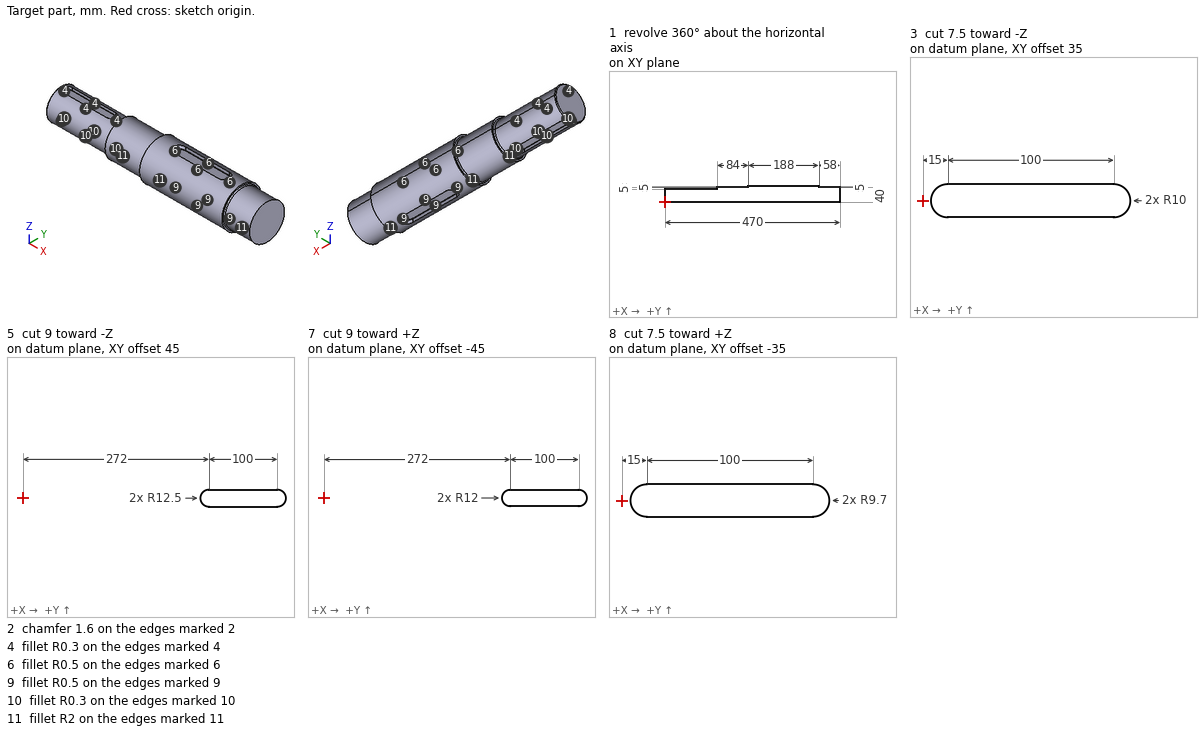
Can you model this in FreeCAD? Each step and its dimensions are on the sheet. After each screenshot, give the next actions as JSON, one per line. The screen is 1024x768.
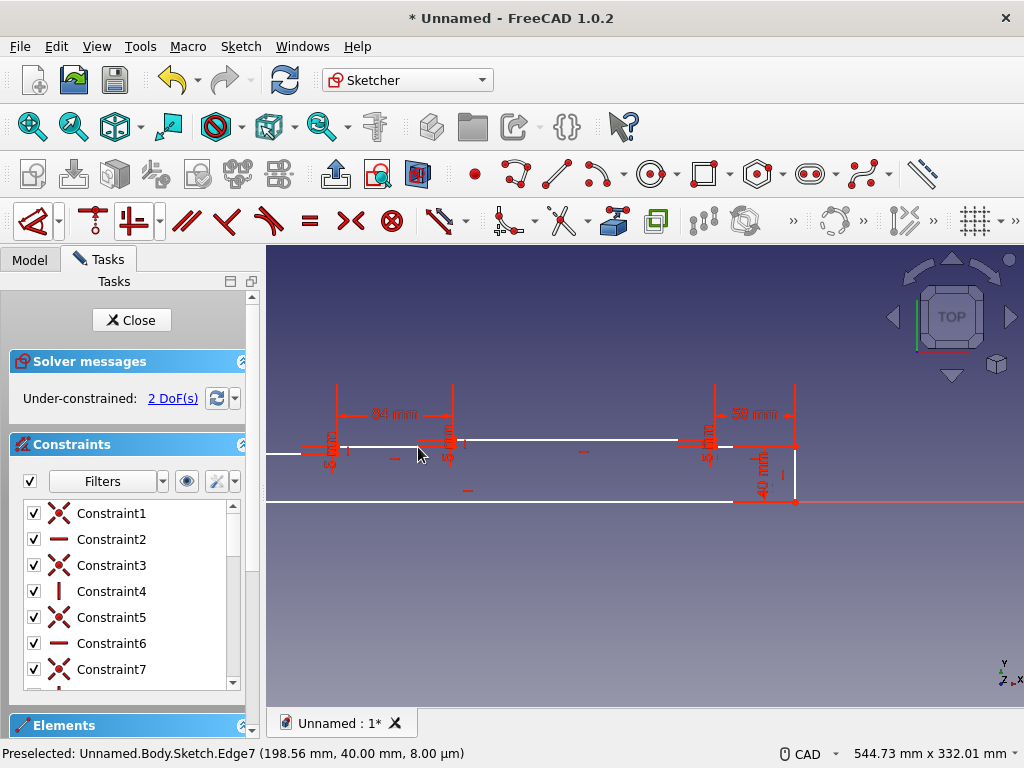
{"action": "left_click", "coordinate": [338, 502]}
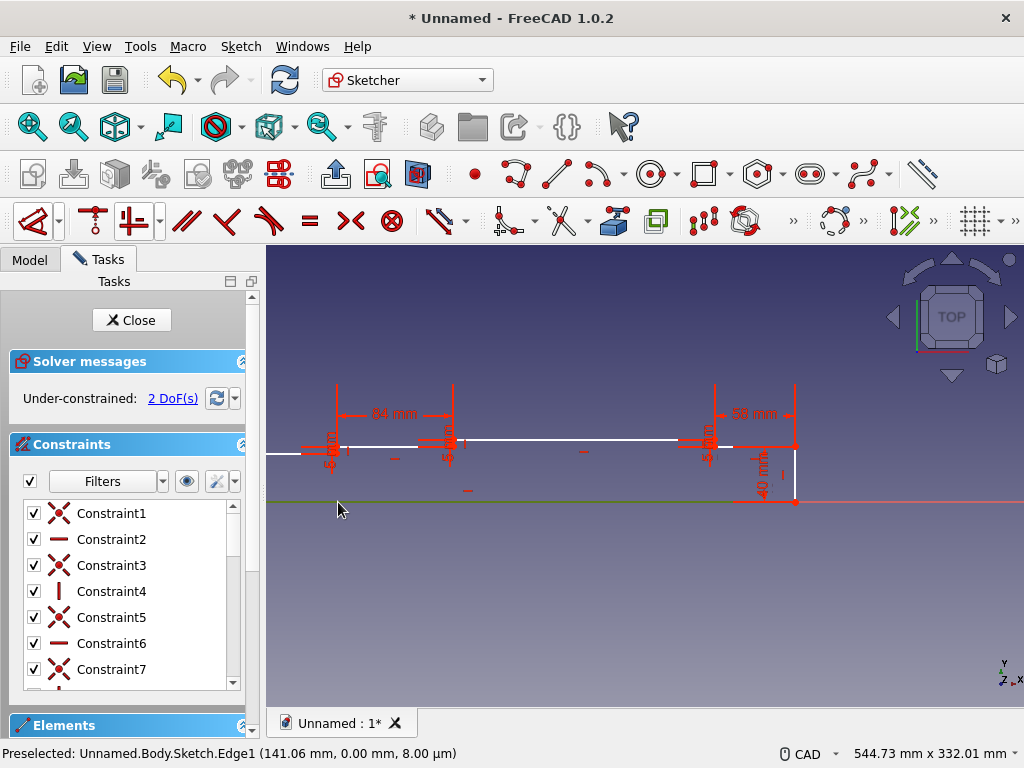
{"action": "left_click", "coordinate": [58, 222]}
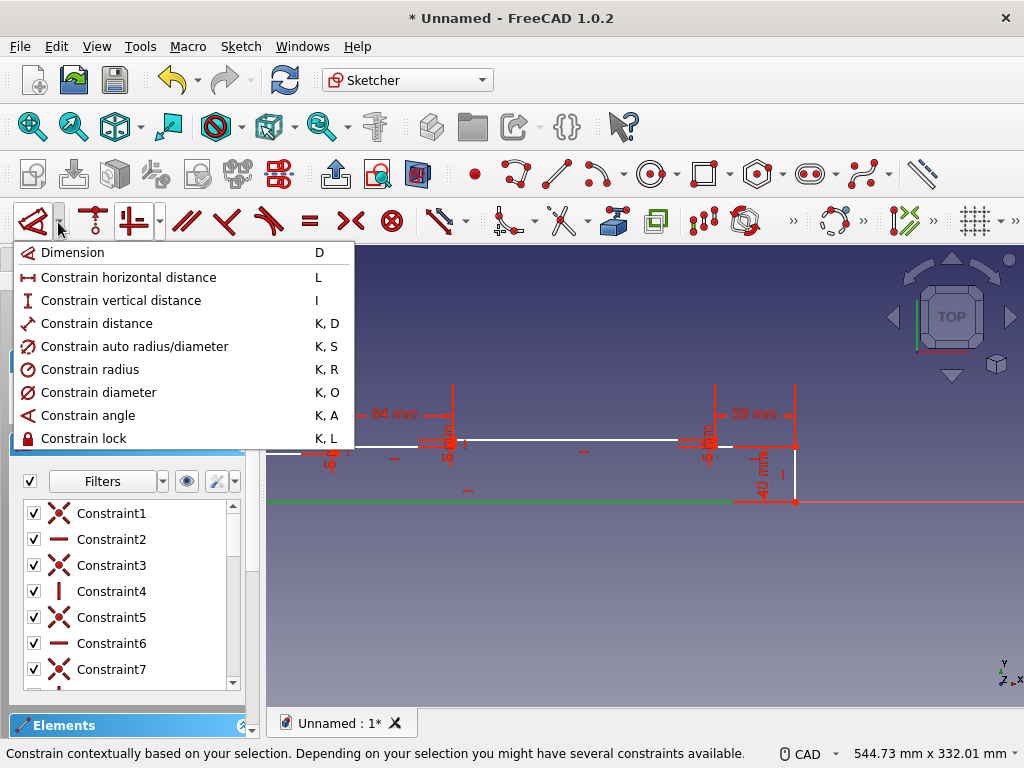
{"action": "left_click", "coordinate": [184, 278]}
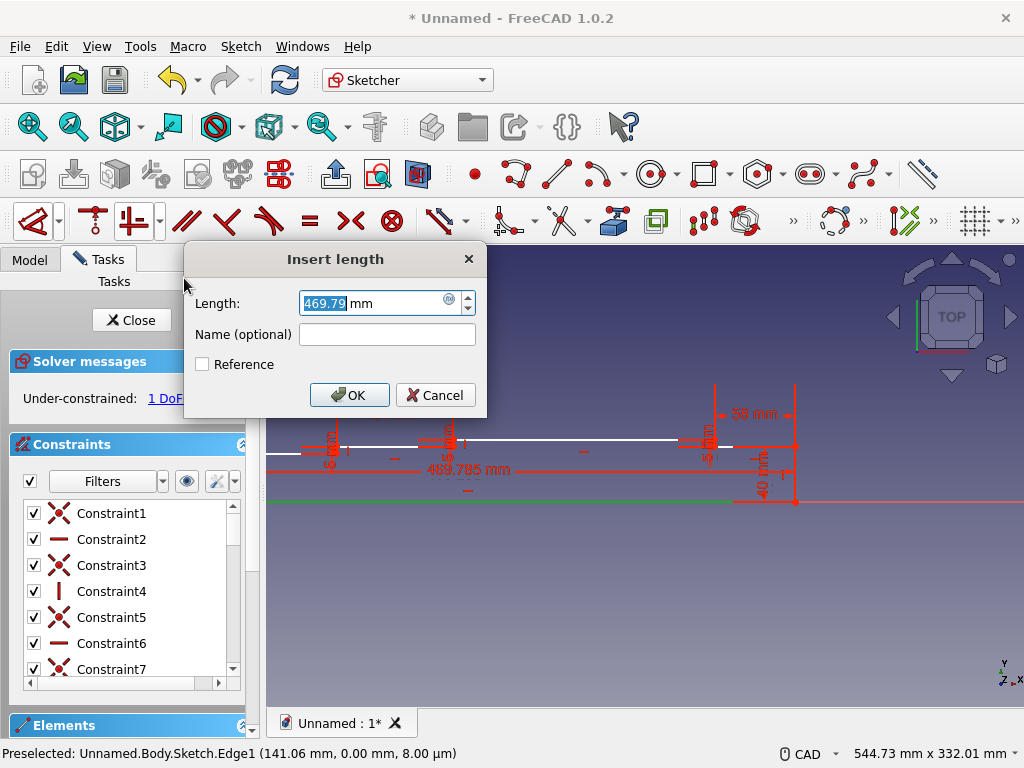
{"action": "type", "text": "470"}
{"action": "key", "text": "Return"}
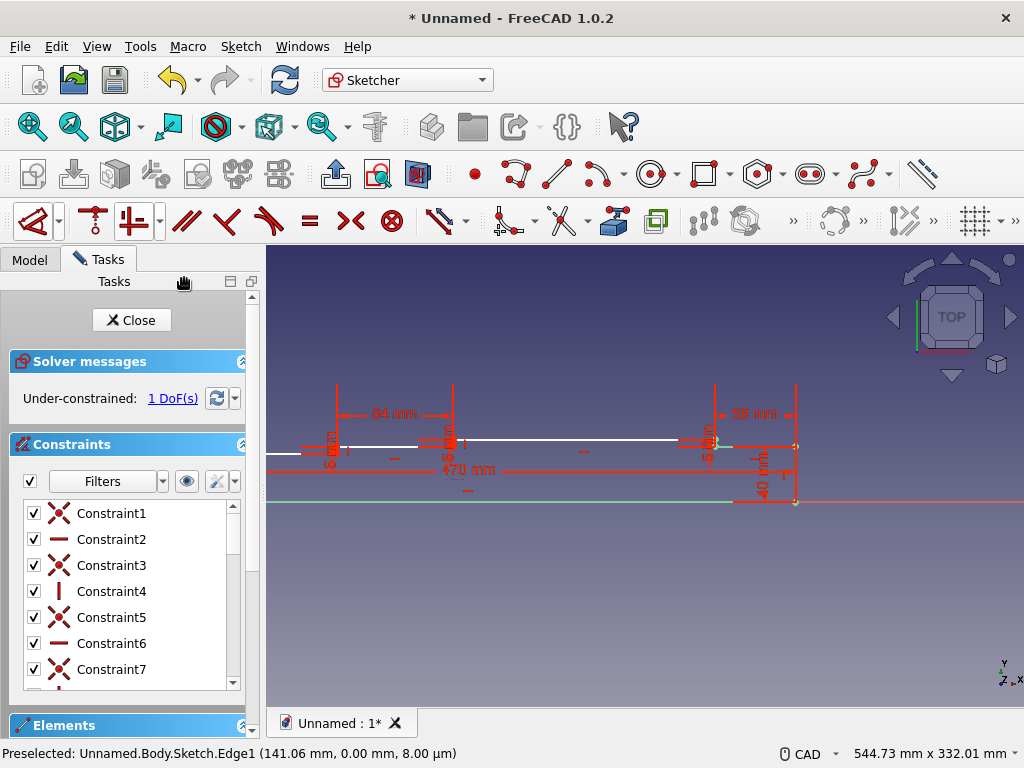
{"action": "left_click", "coordinate": [637, 440]}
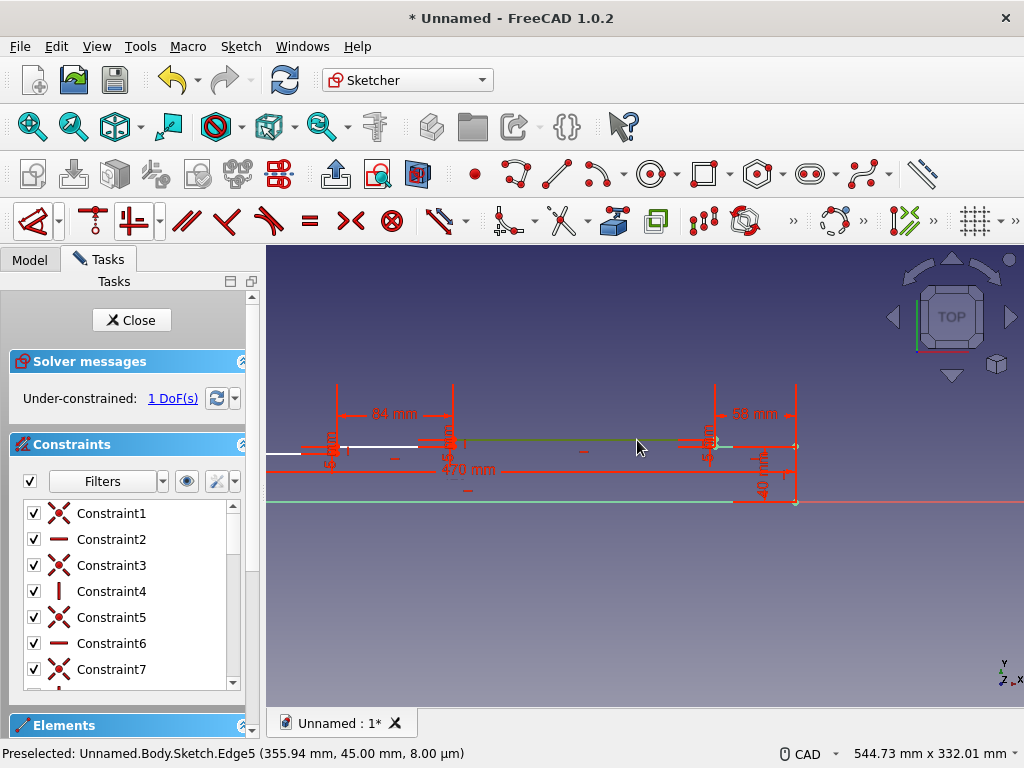
{"action": "left_click", "coordinate": [58, 222]}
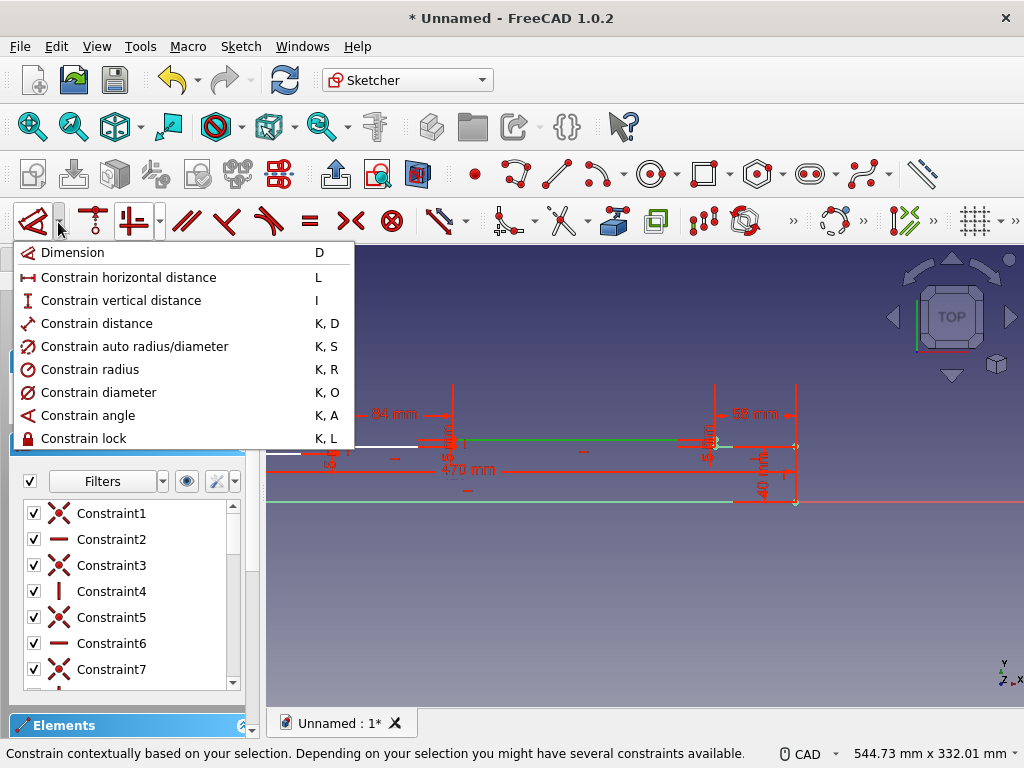
{"action": "left_click", "coordinate": [184, 278]}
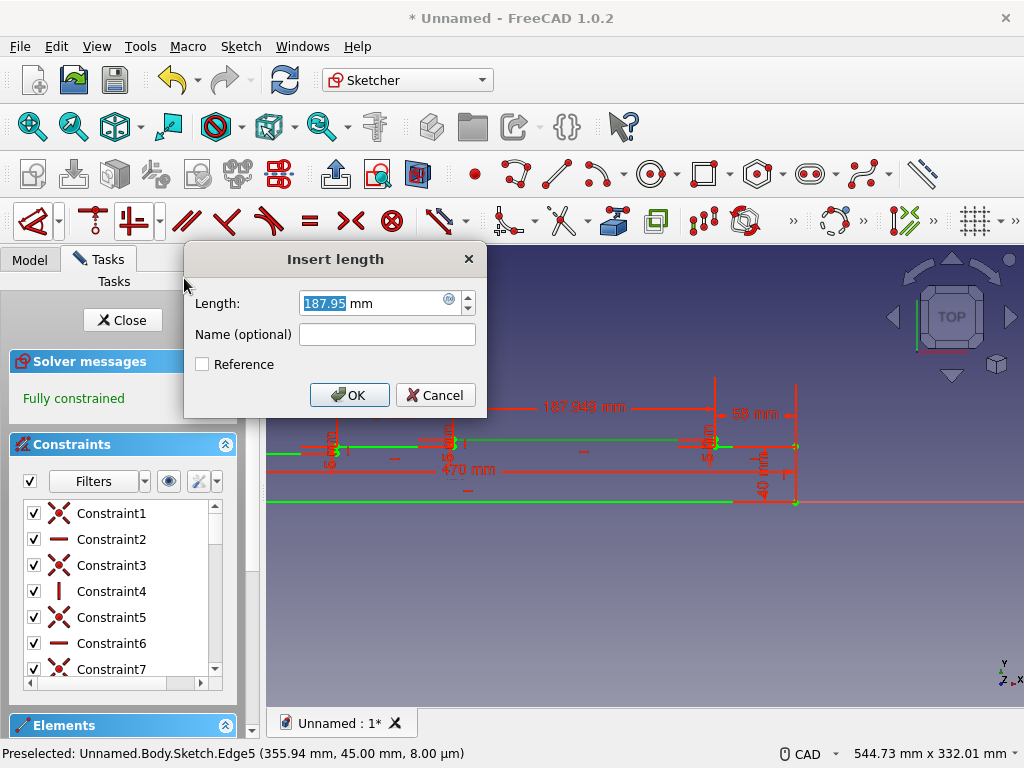
{"action": "type", "text": "188"}
{"action": "key", "text": "Return"}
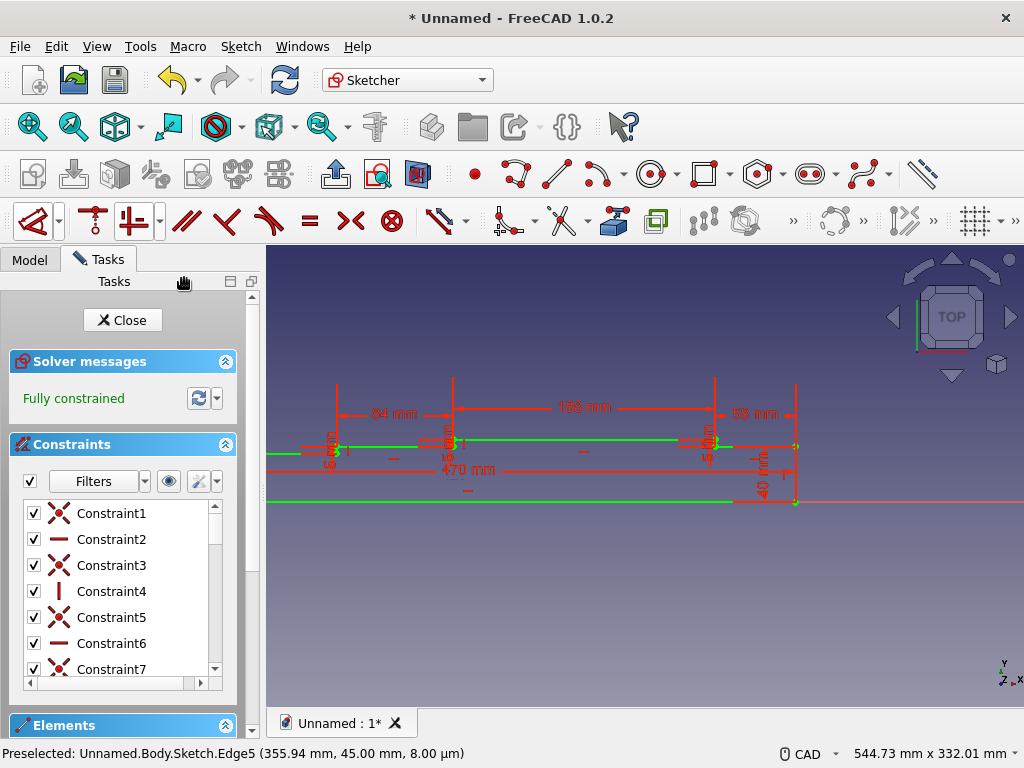
{"action": "left_click", "coordinate": [123, 320]}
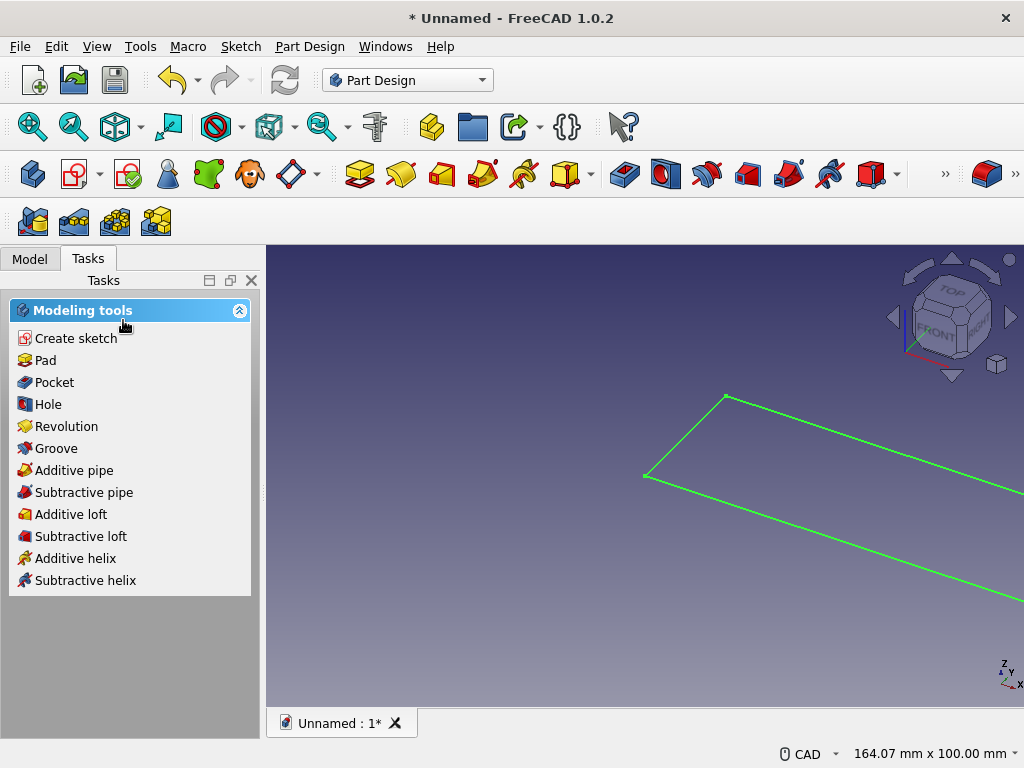
{"action": "left_click", "coordinate": [401, 174]}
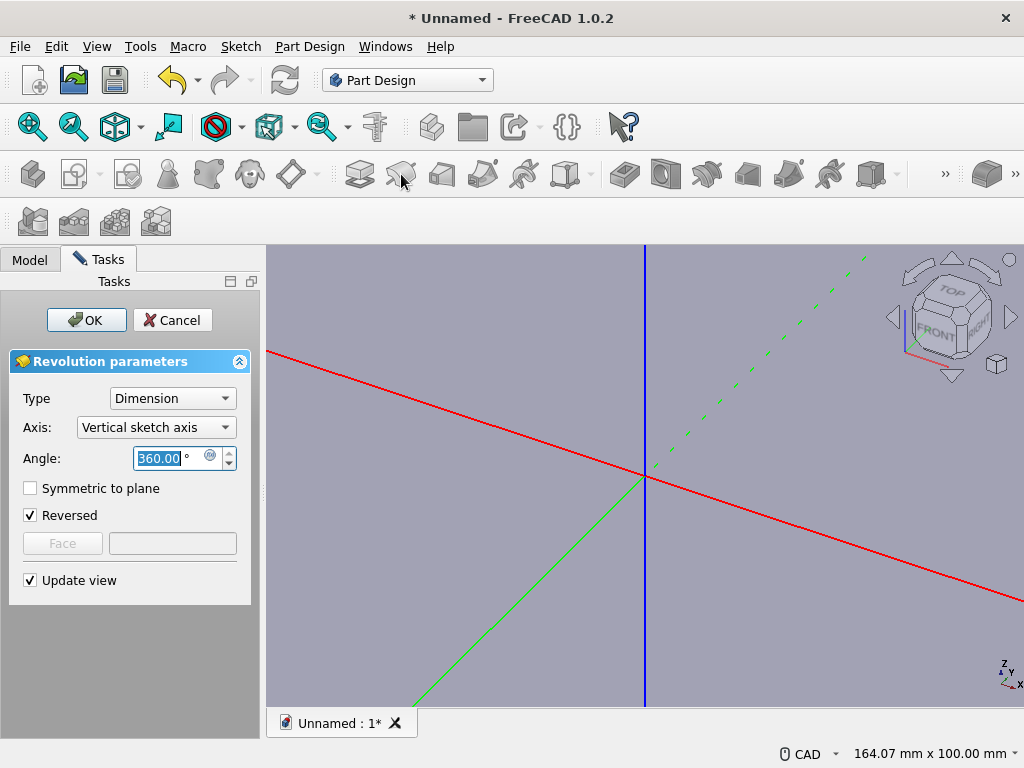
{"action": "left_click", "coordinate": [157, 428]}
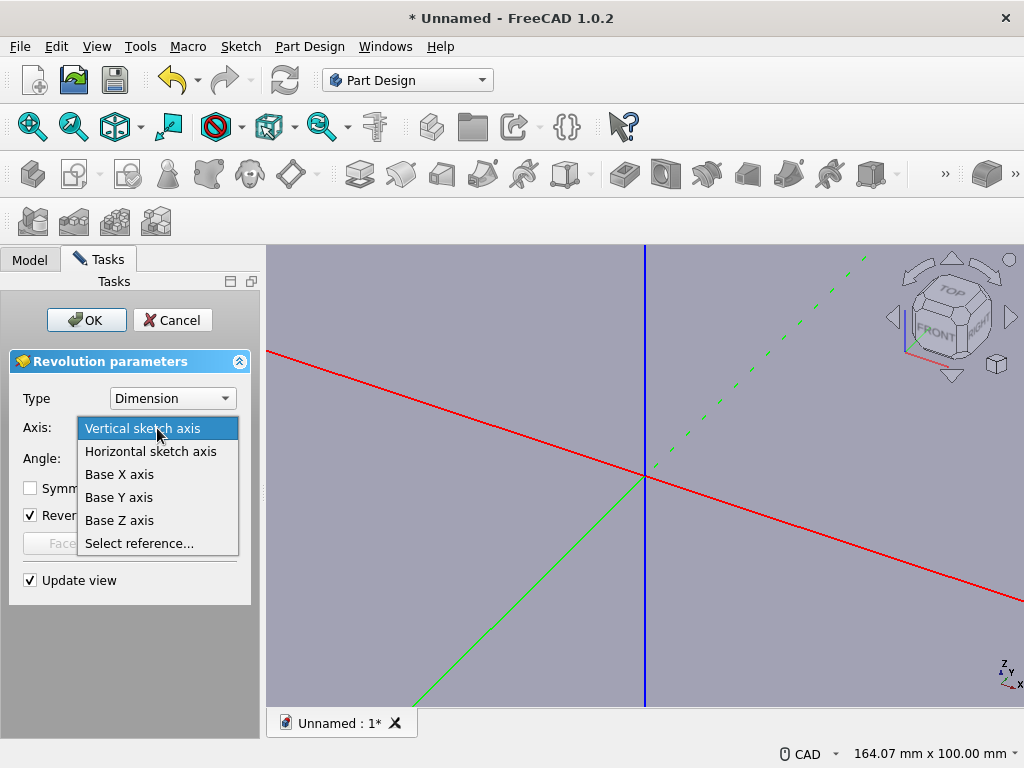
{"action": "left_click", "coordinate": [156, 452]}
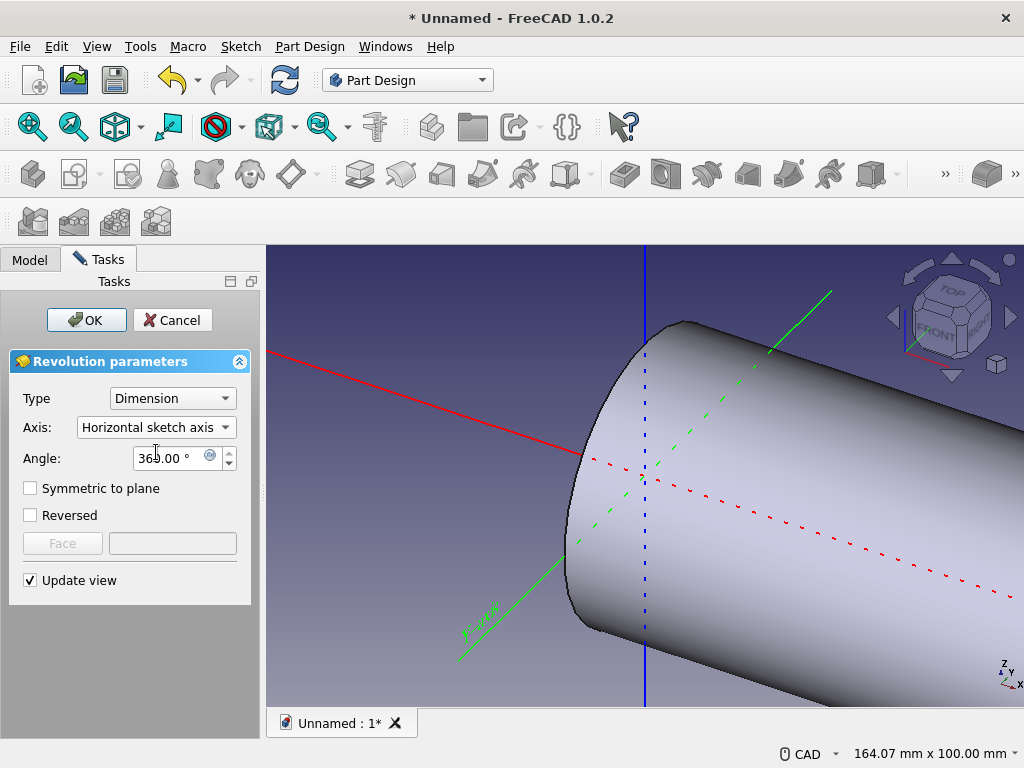
{"action": "left_click", "coordinate": [87, 320]}